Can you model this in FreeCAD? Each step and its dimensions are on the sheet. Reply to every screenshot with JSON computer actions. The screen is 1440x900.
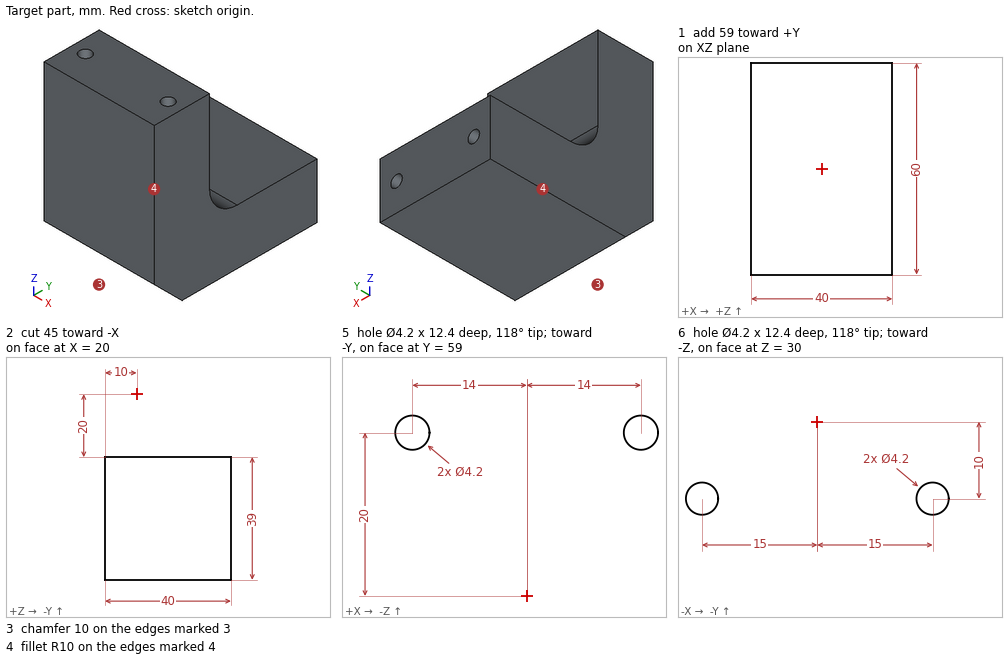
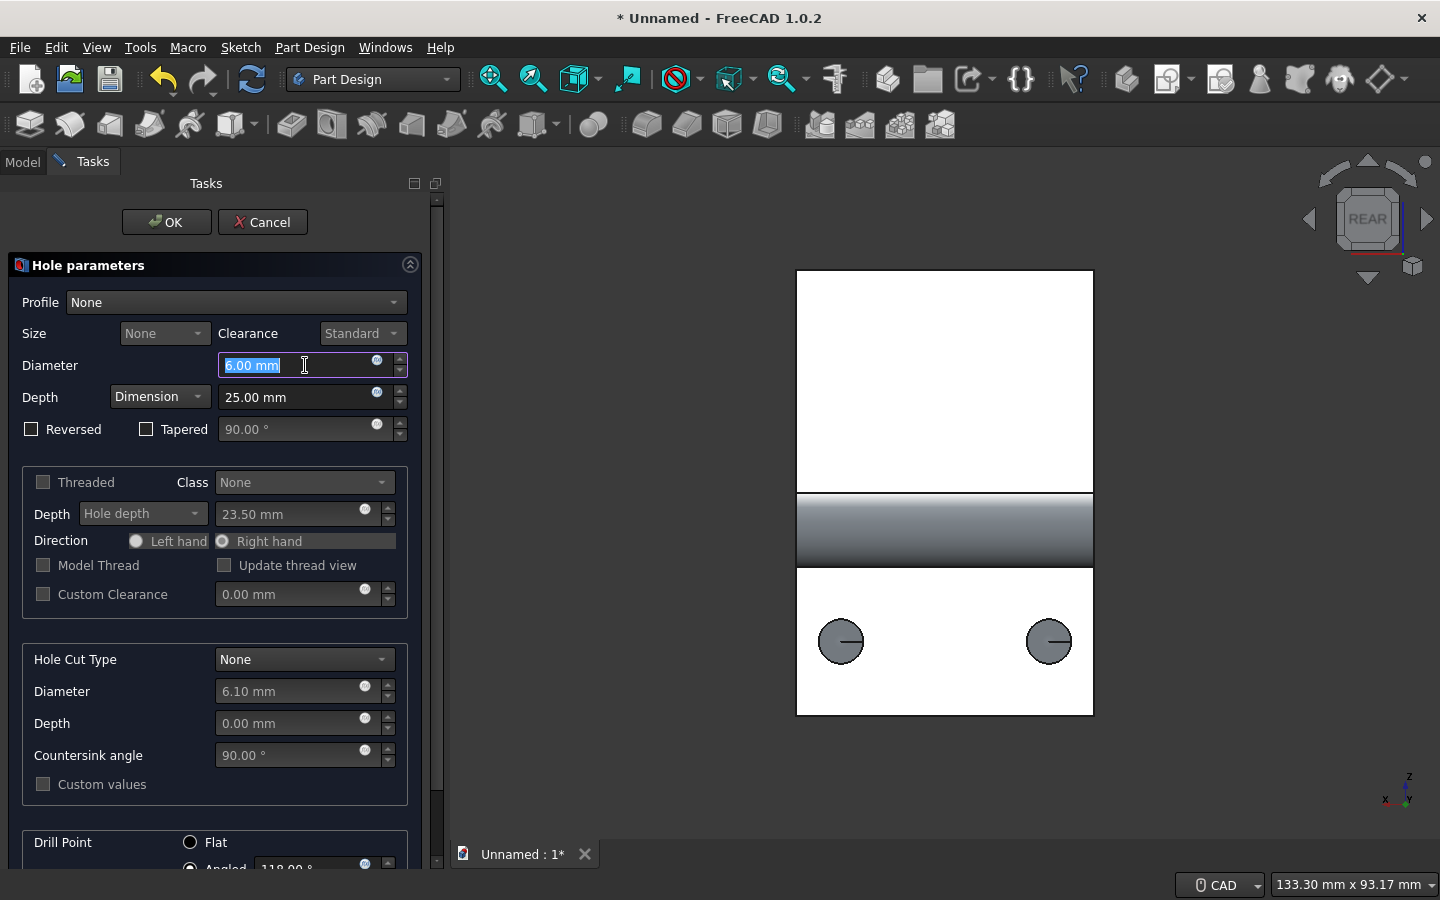
{"action": "type", "text": "4.2"}
{"action": "key", "text": "Tab"}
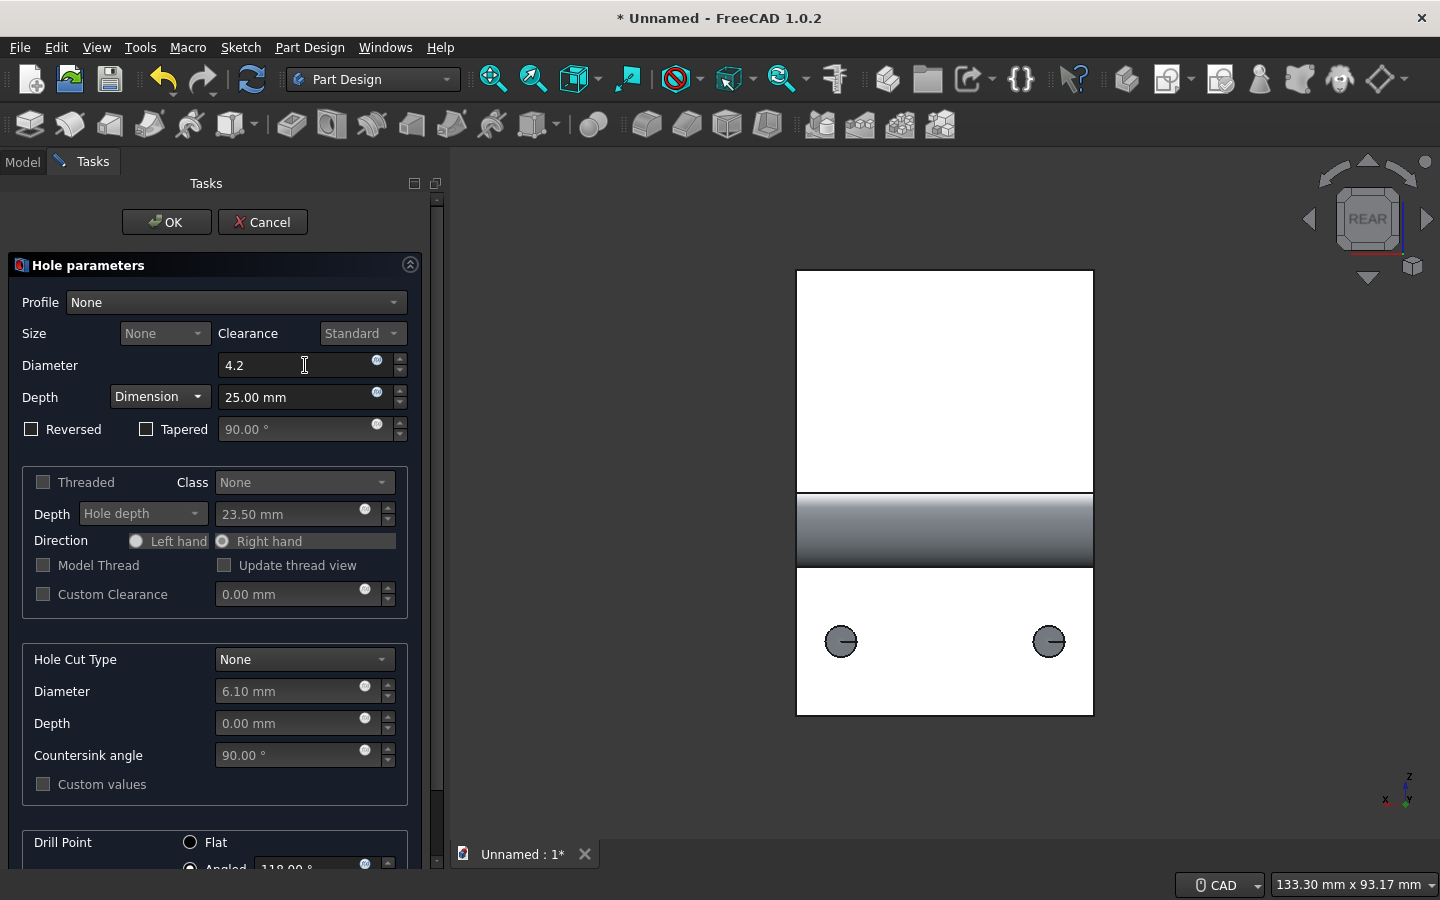
{"action": "triple_click", "coordinate": [305, 397]}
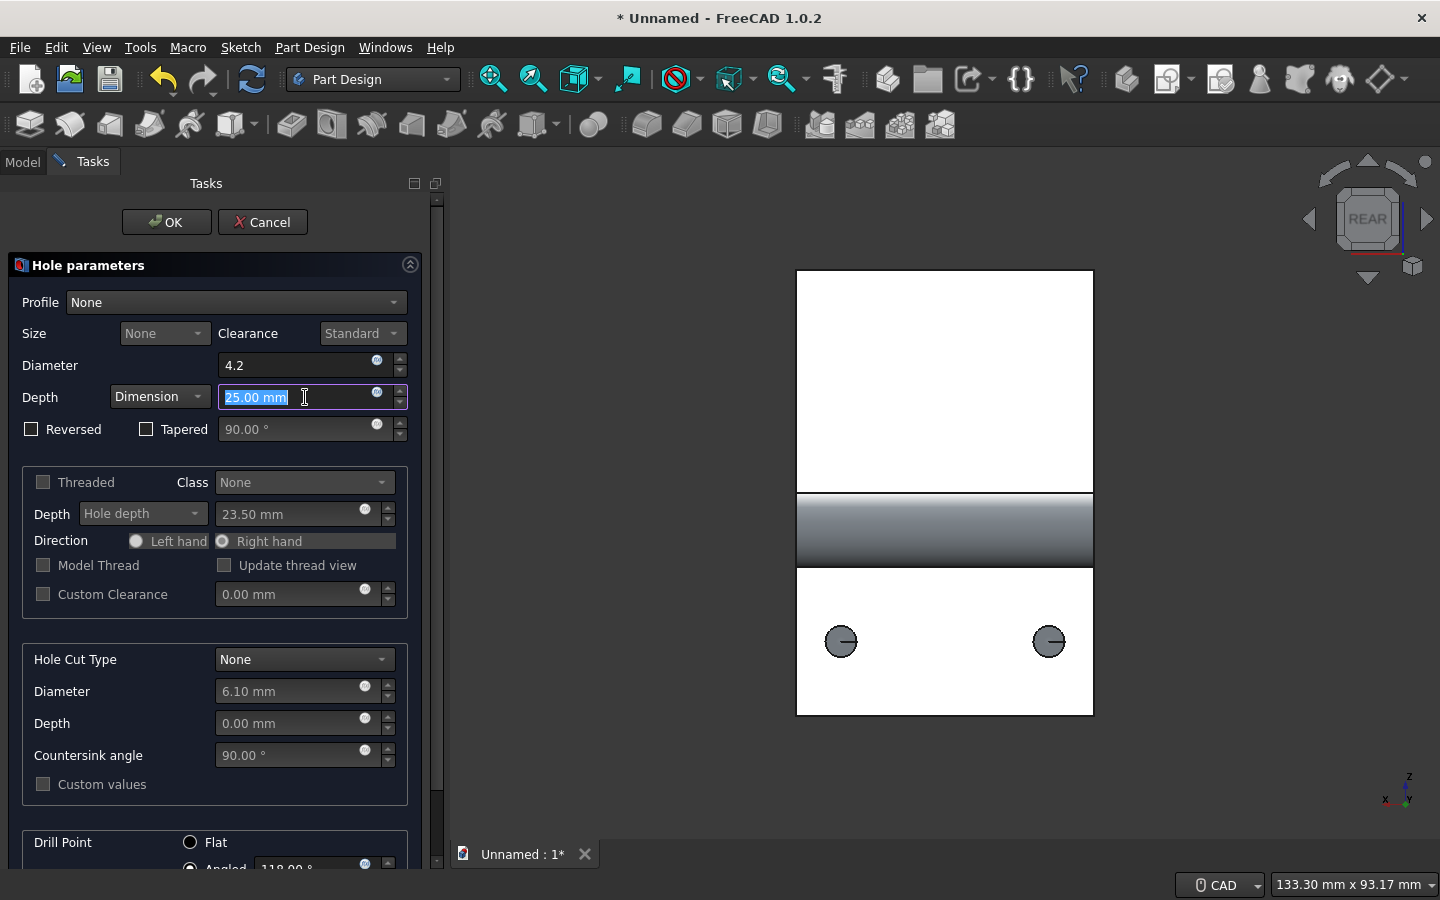
{"action": "type", "text": "12.4"}
{"action": "key", "text": "Tab"}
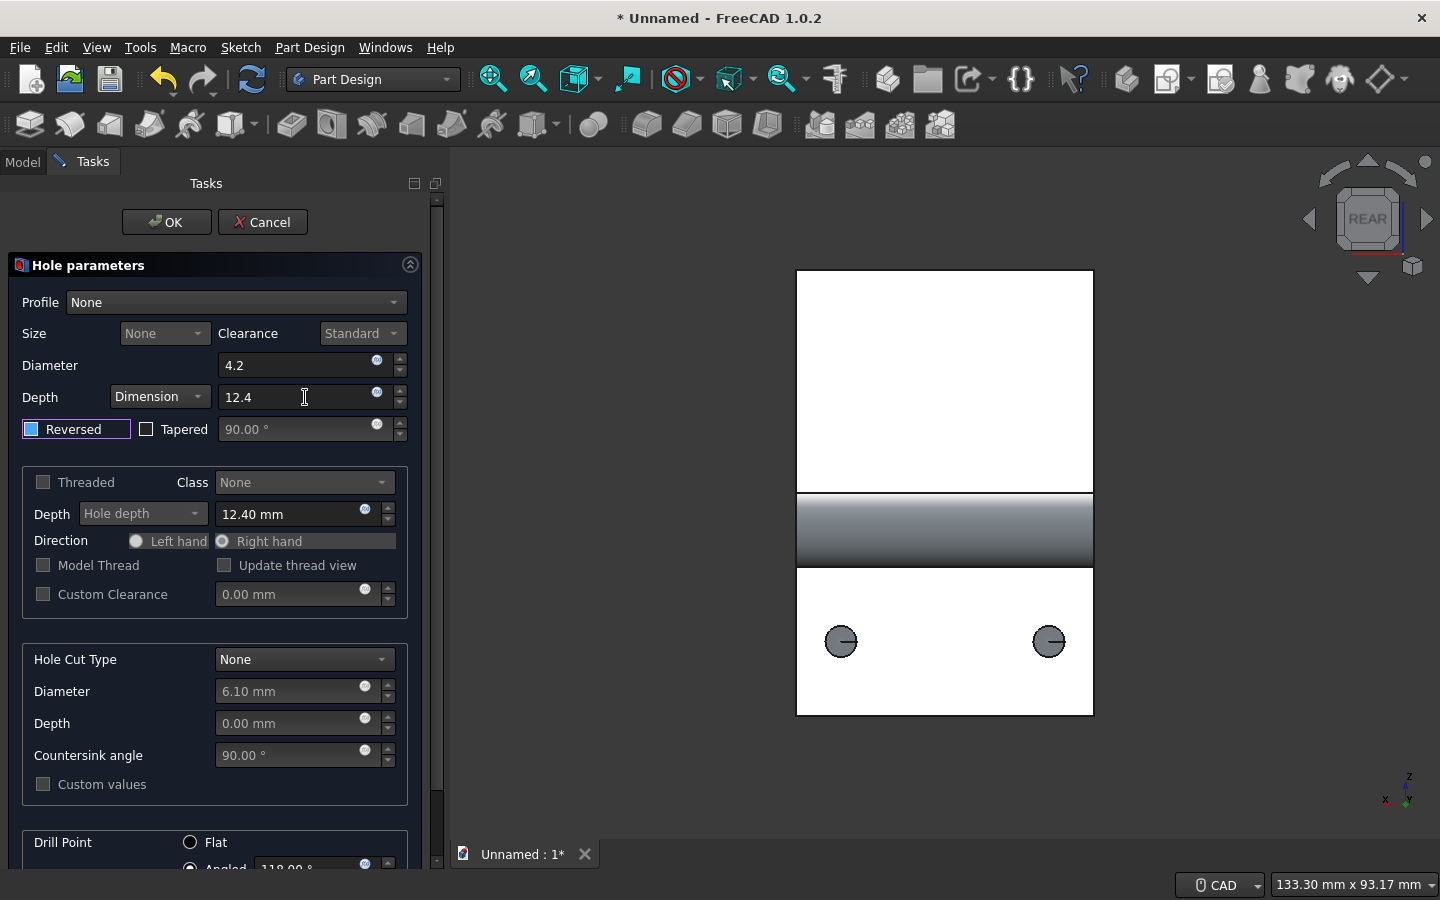
{"action": "left_click", "coordinate": [167, 222]}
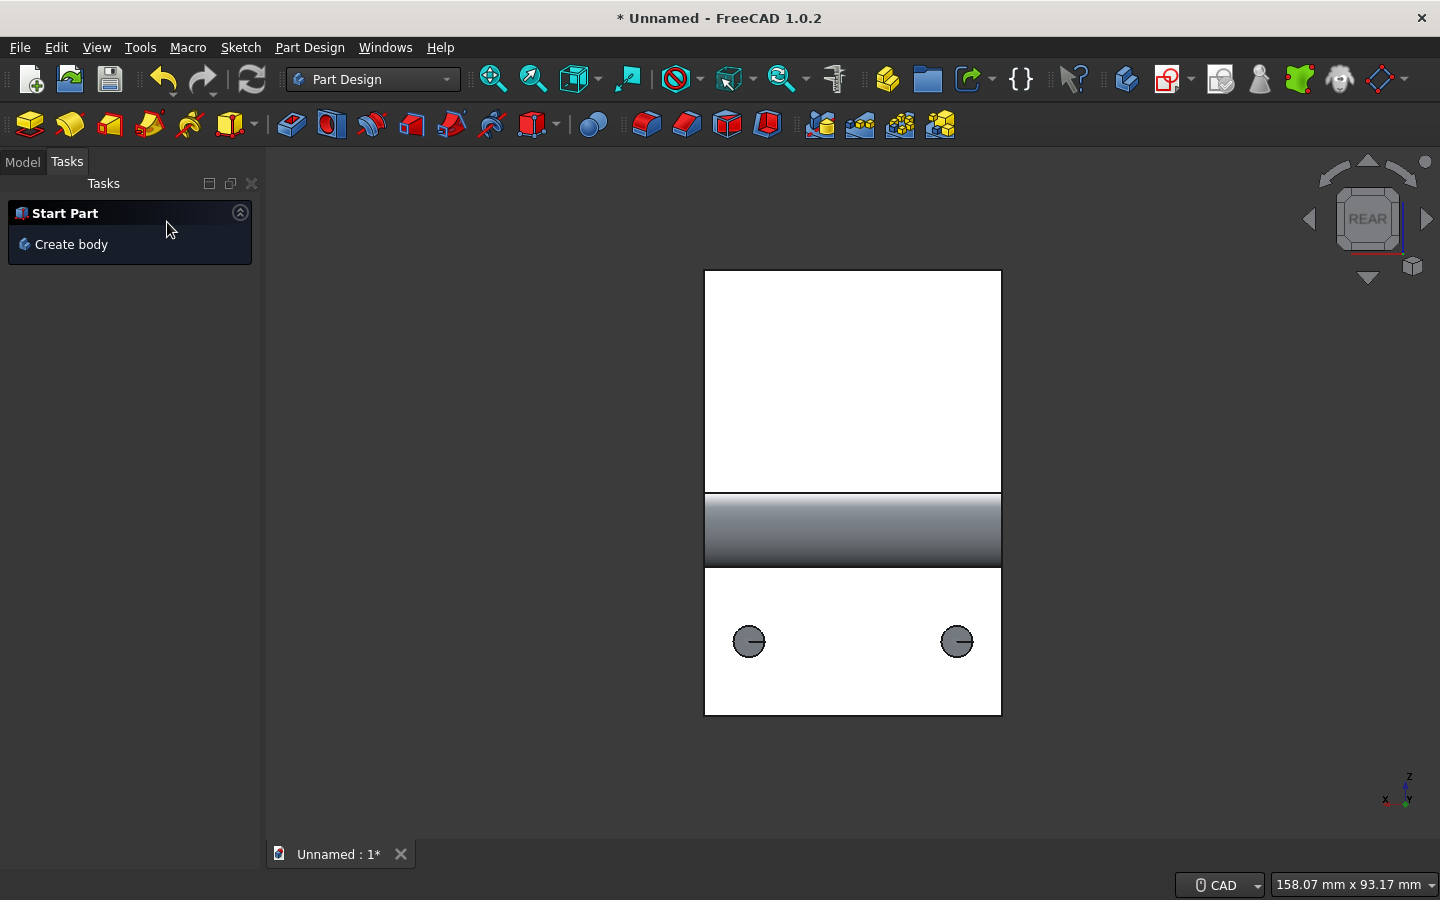
{"action": "key", "text": "0"}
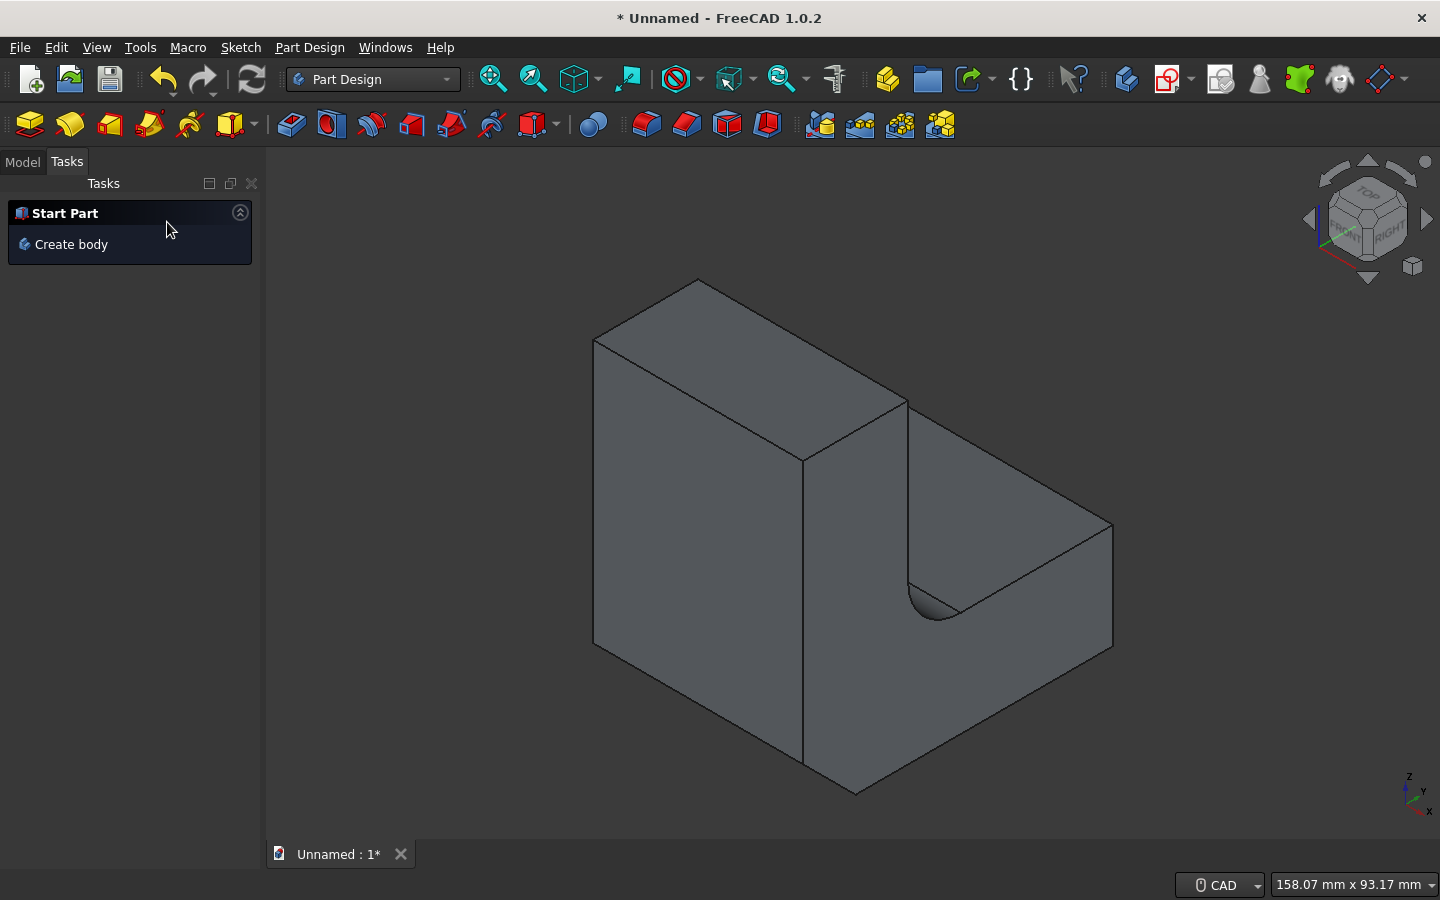
{"action": "left_click", "coordinate": [781, 387]}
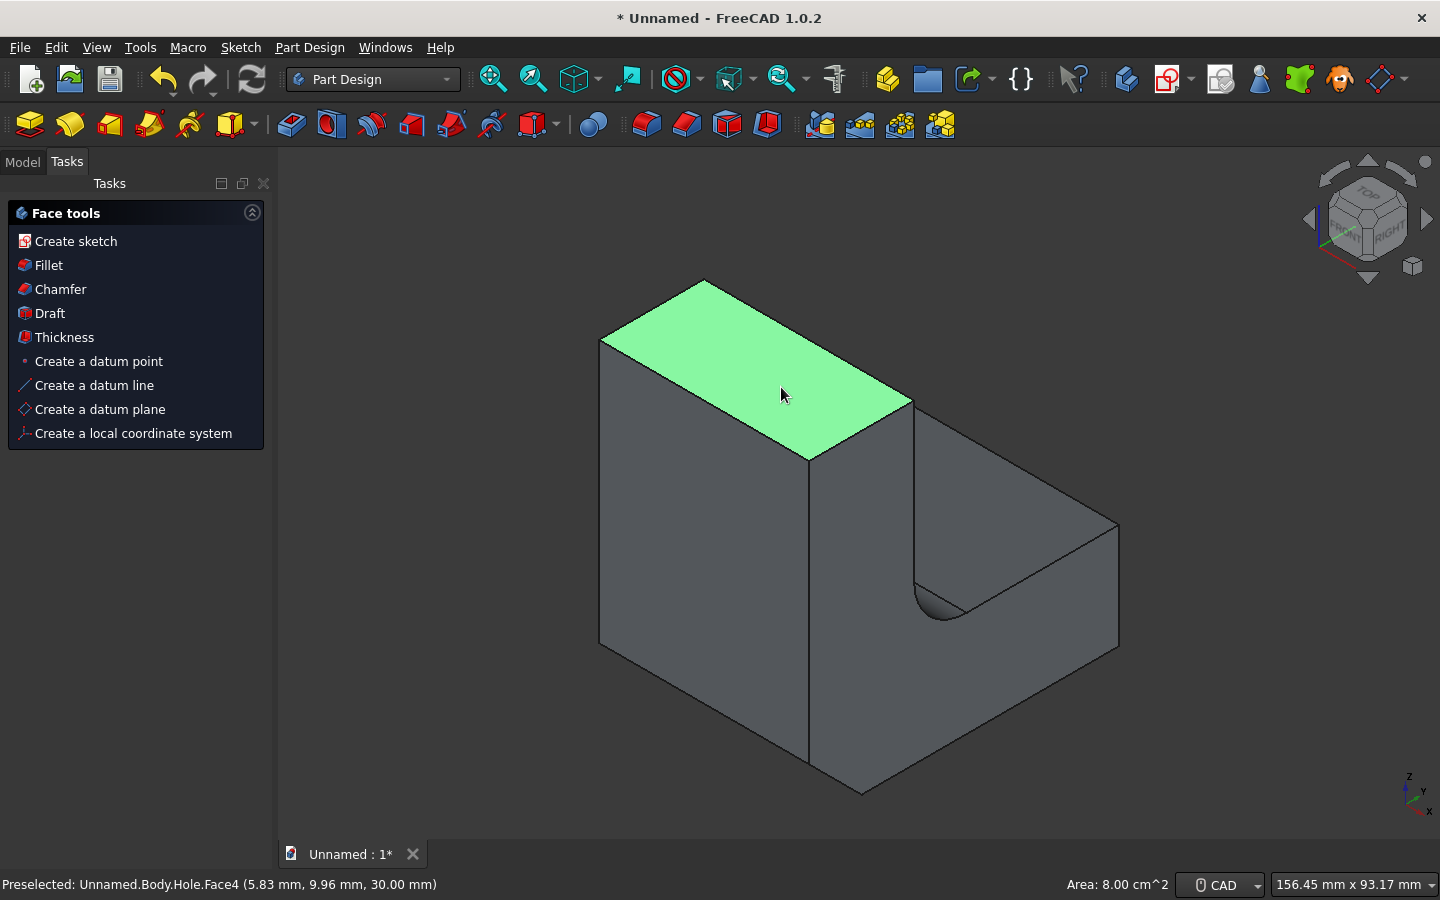
{"action": "left_click", "coordinate": [1168, 80]}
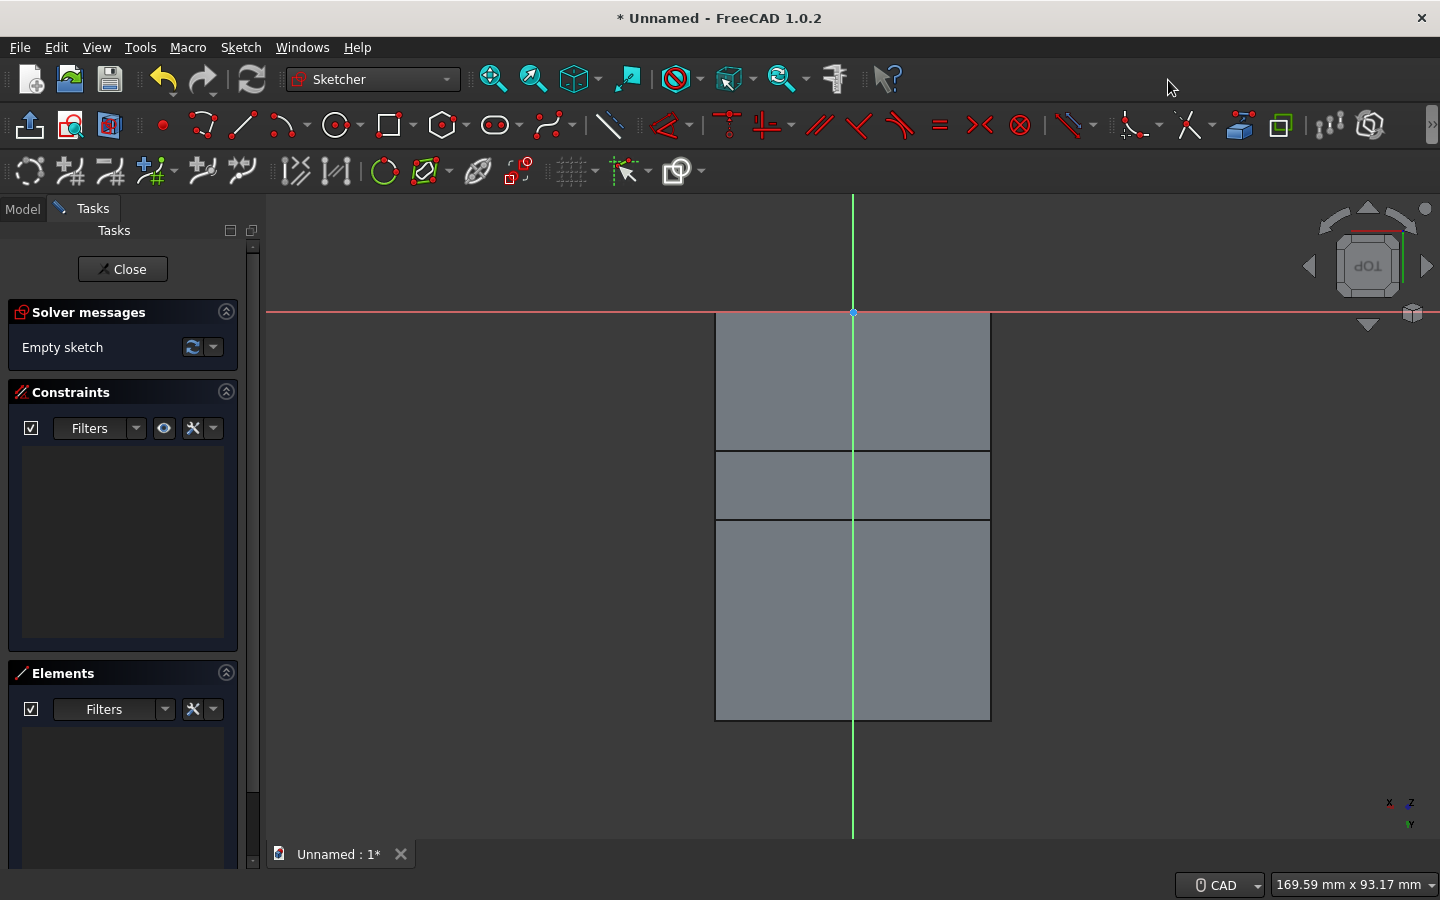
{"action": "scroll", "coordinate": [893, 260], "scroll_direction": "up", "scroll_amount": 5}